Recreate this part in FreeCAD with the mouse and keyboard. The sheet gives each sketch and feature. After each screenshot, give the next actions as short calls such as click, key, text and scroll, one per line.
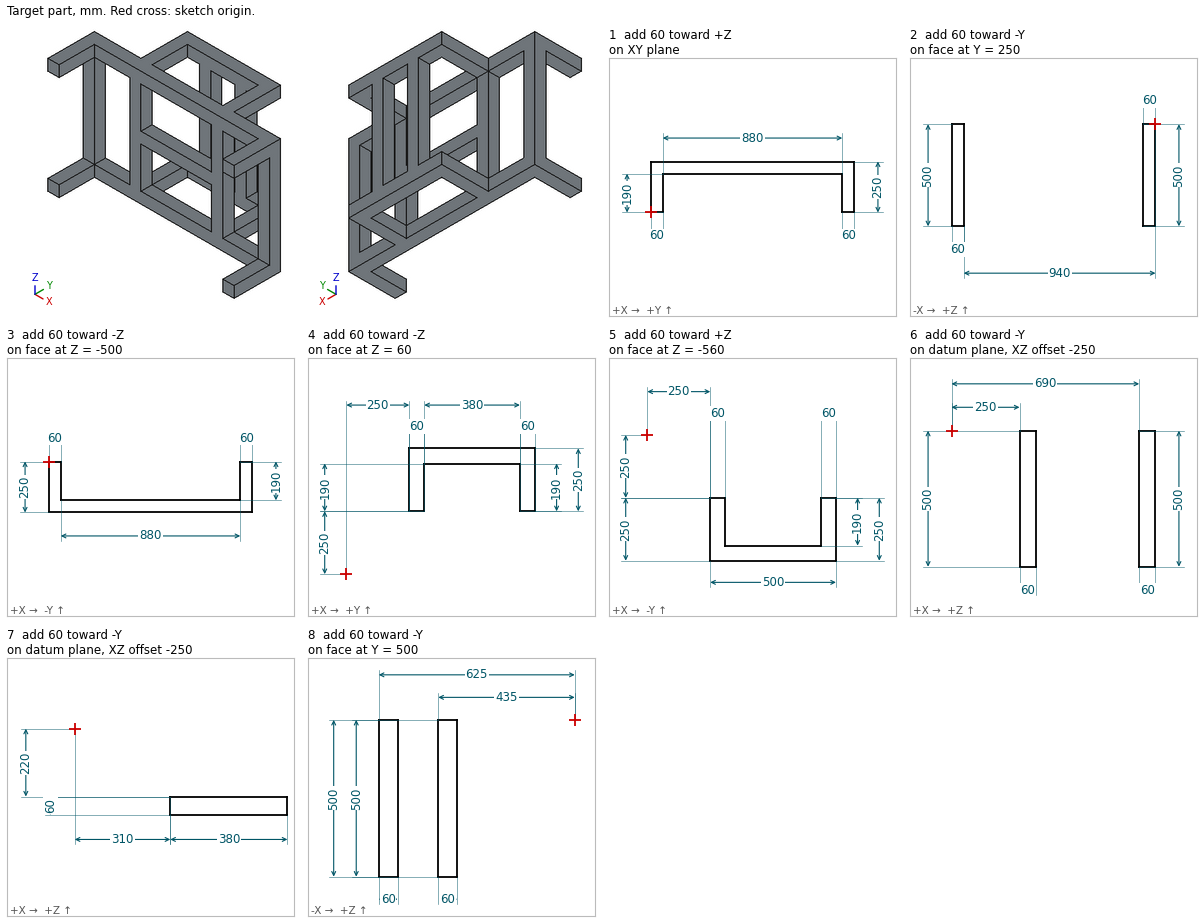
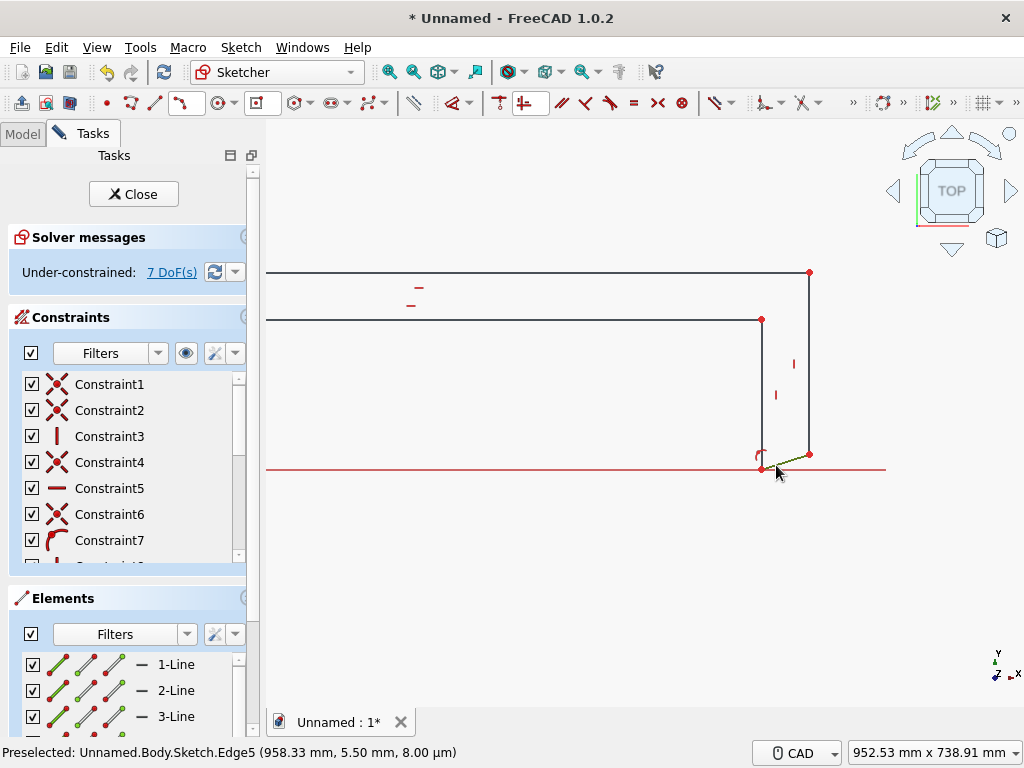
click(544, 104)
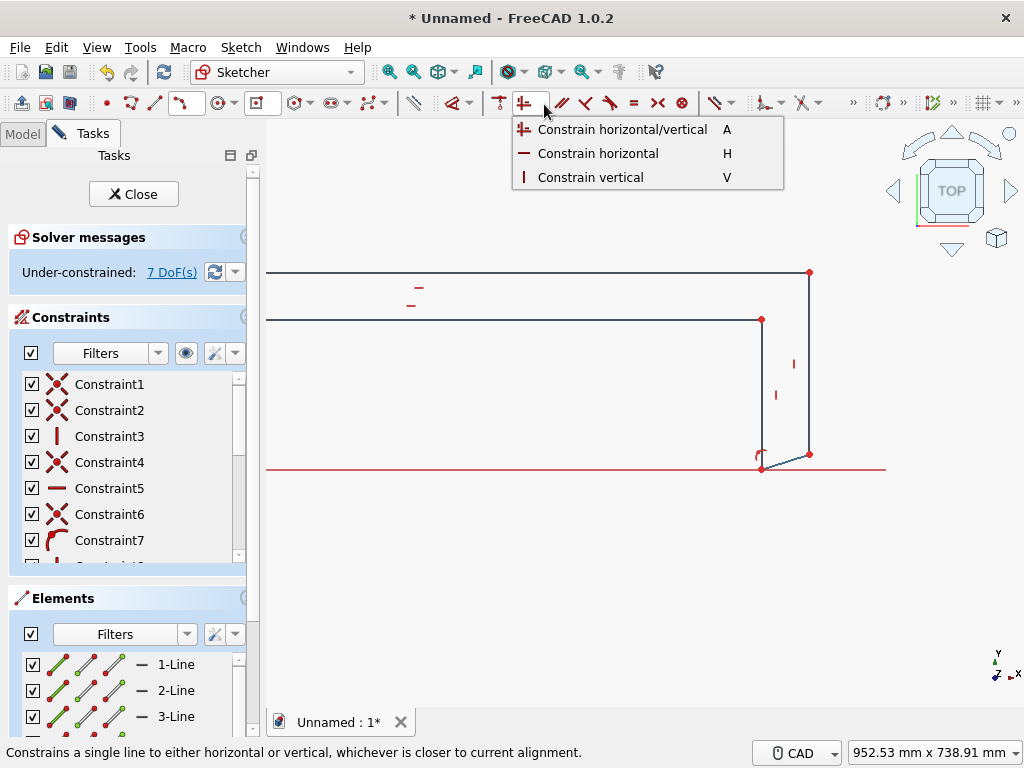
click(648, 153)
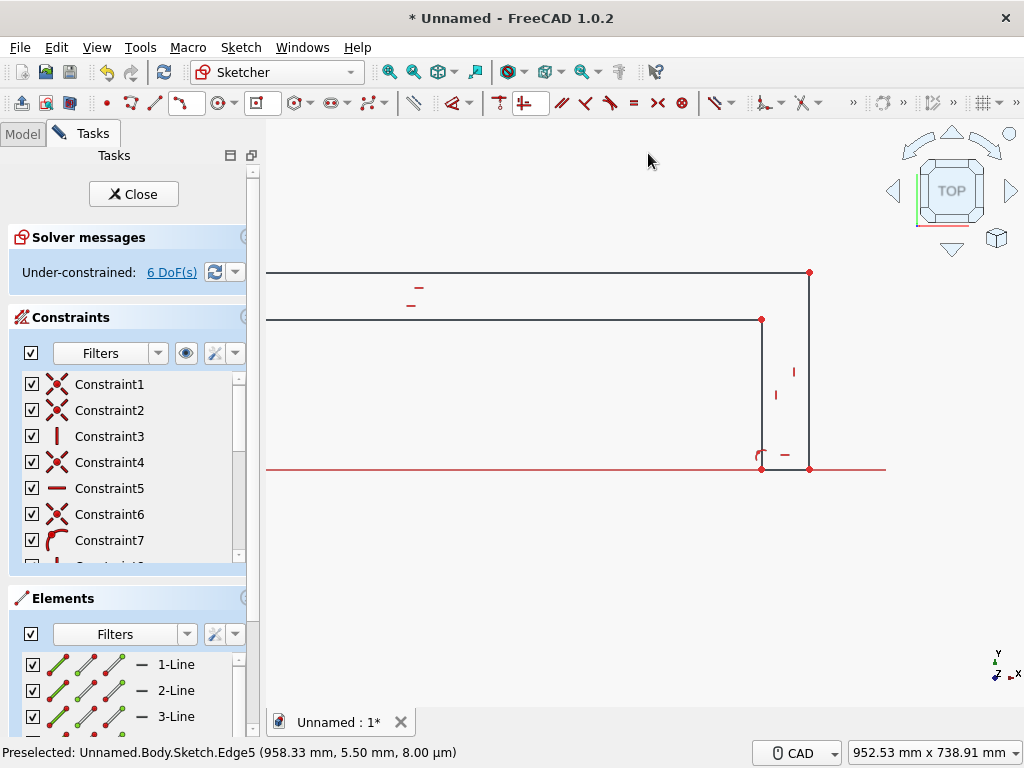
scroll(778, 465, down, 3)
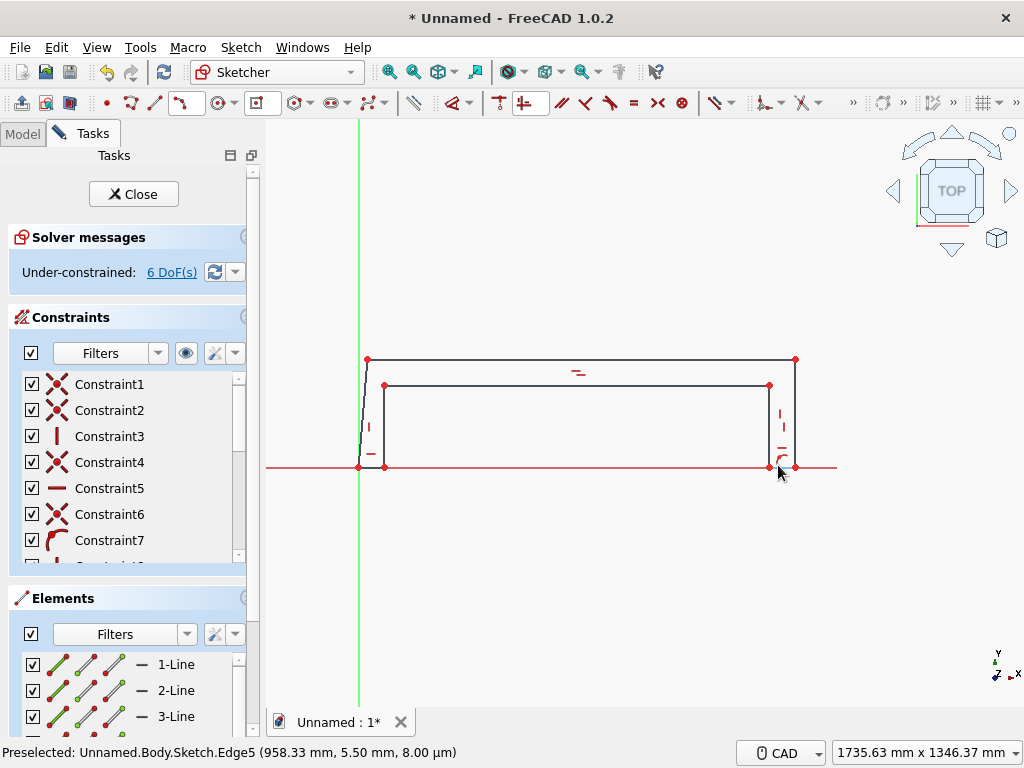
scroll(365, 392, up, 4)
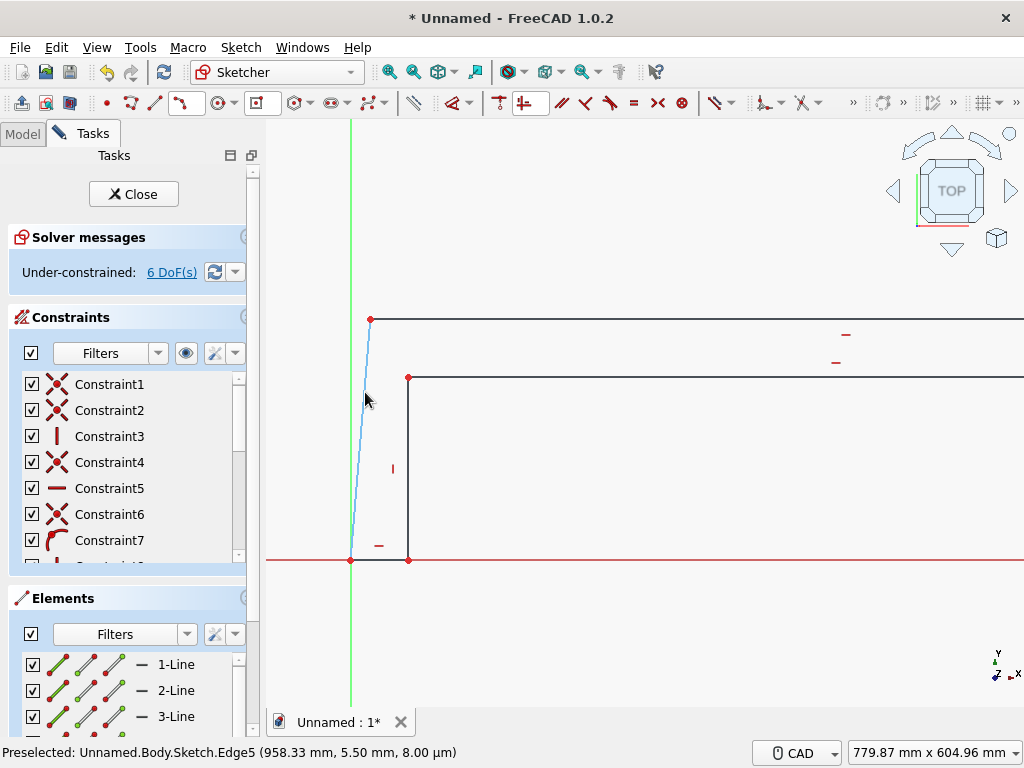
click(364, 392)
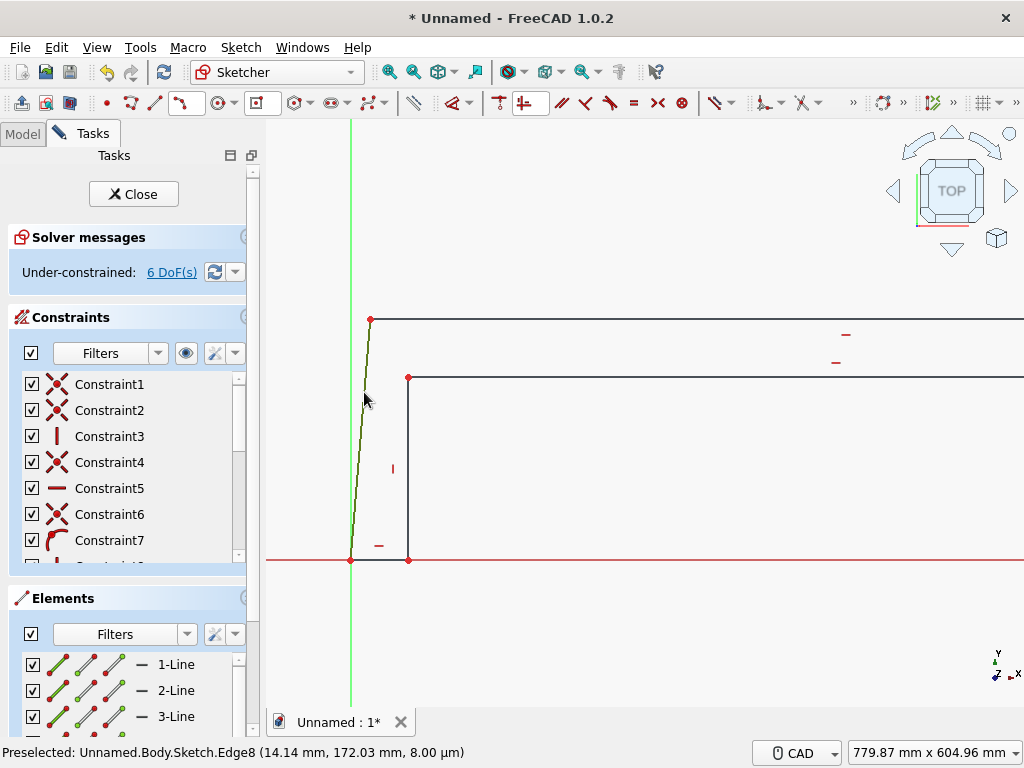
key(v)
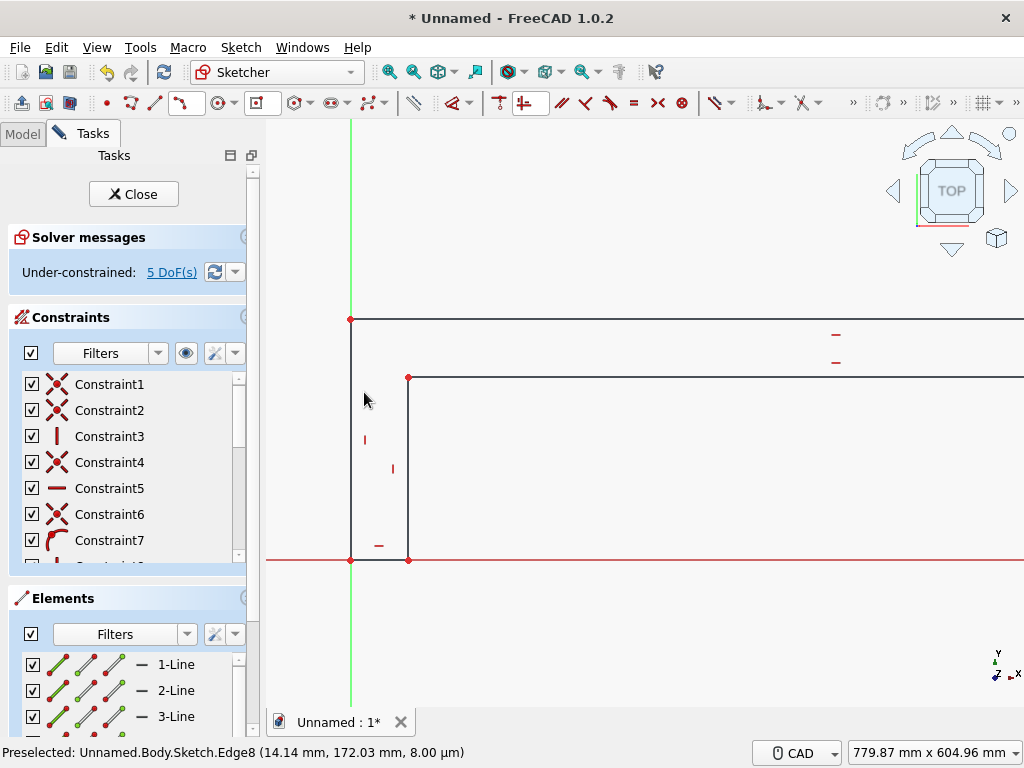
click(452, 104)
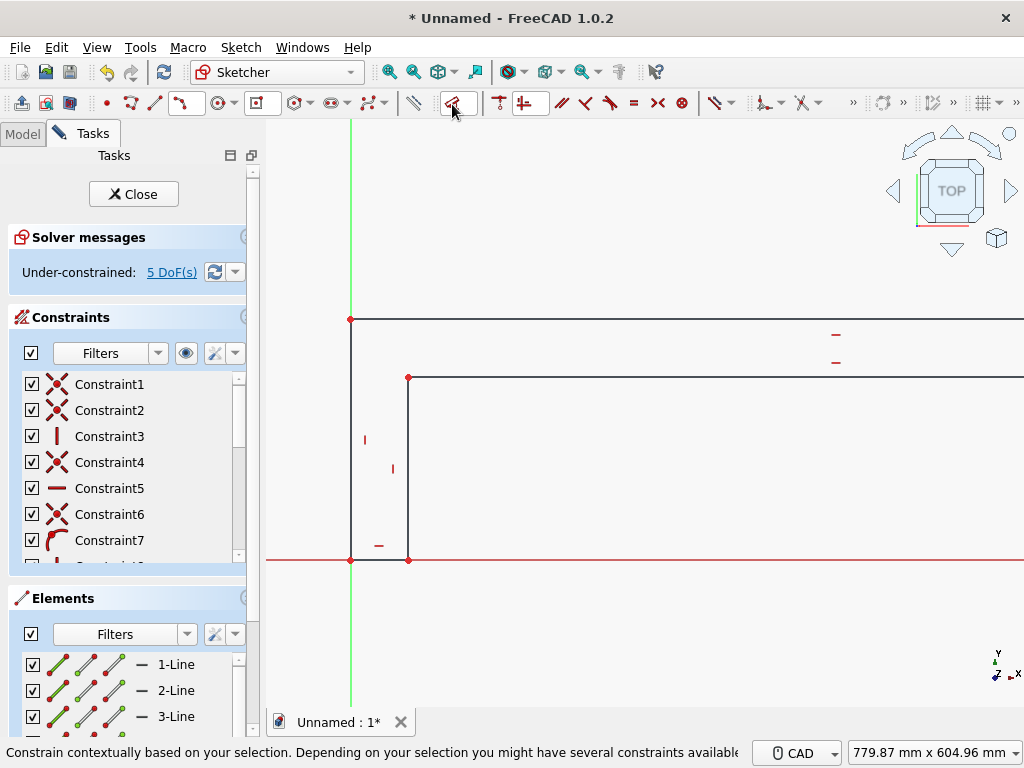
click(368, 560)
click(379, 594)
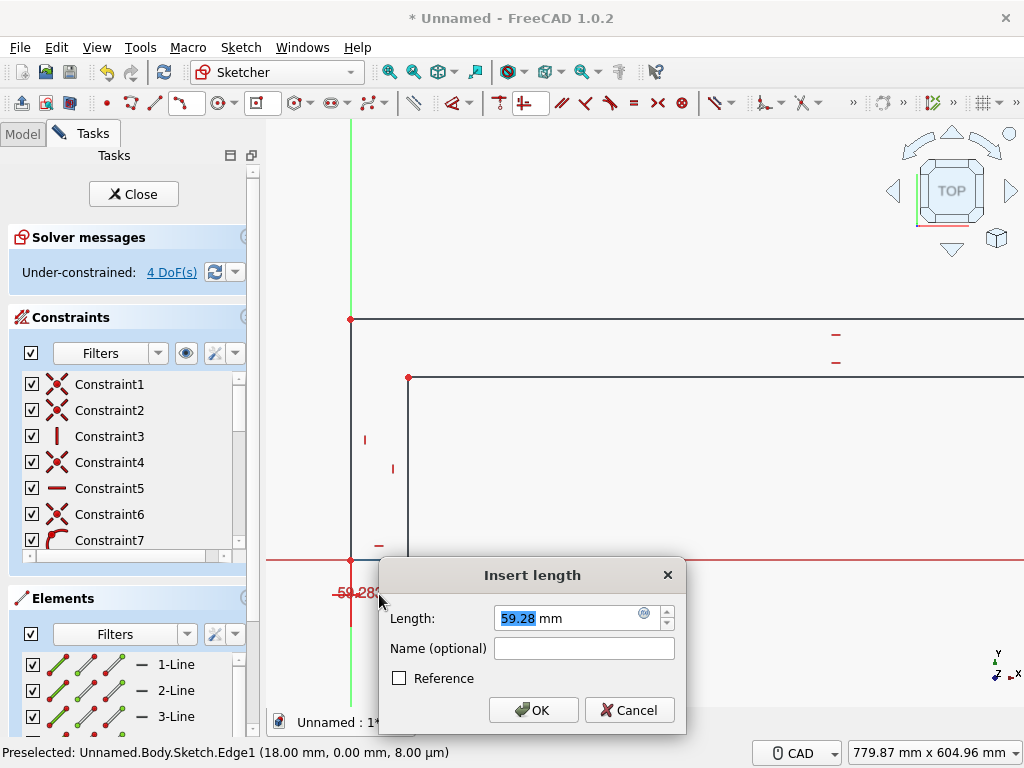
text(60)
key(Return)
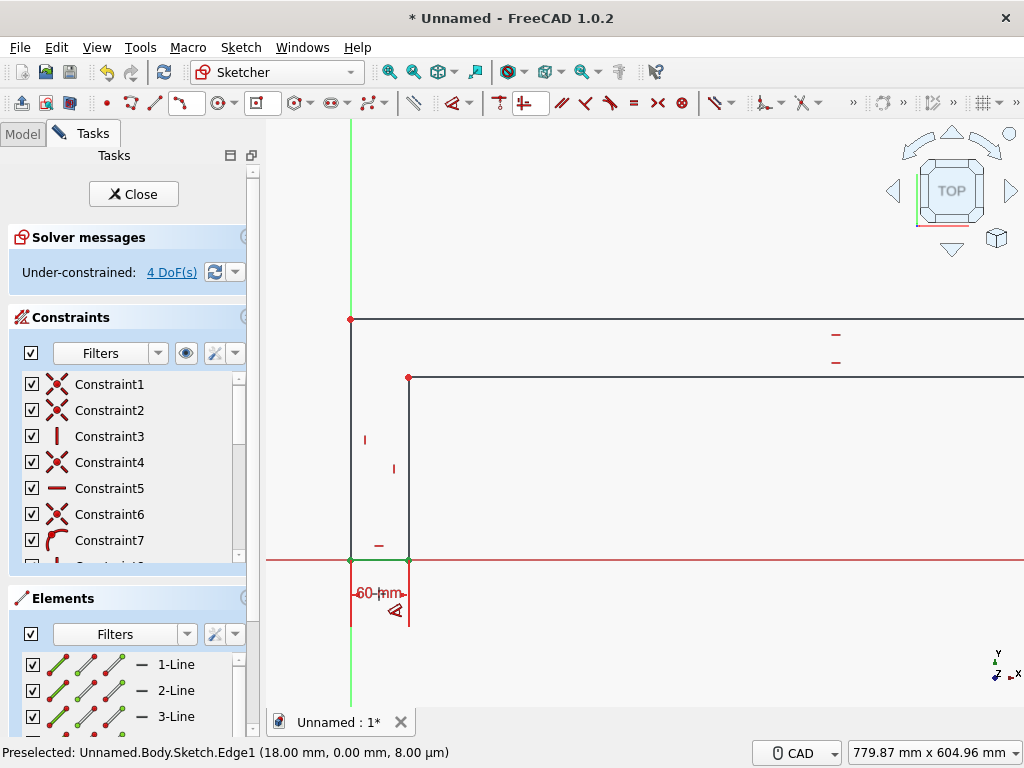
scroll(364, 392, down, 4)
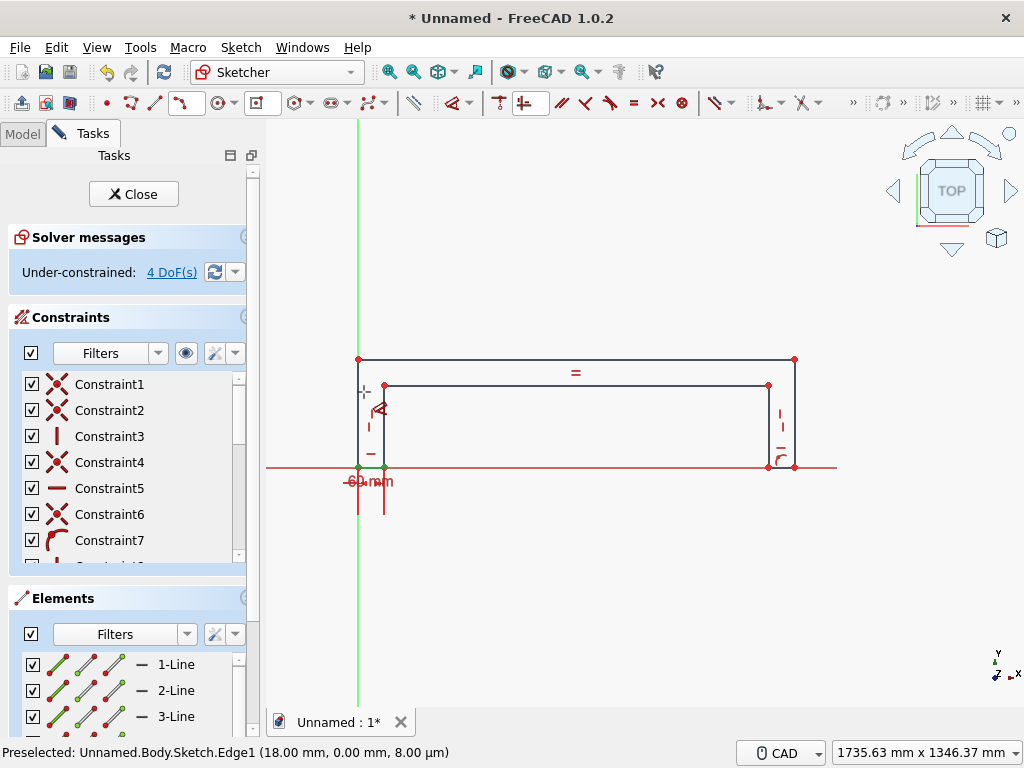
scroll(777, 468, up, 3)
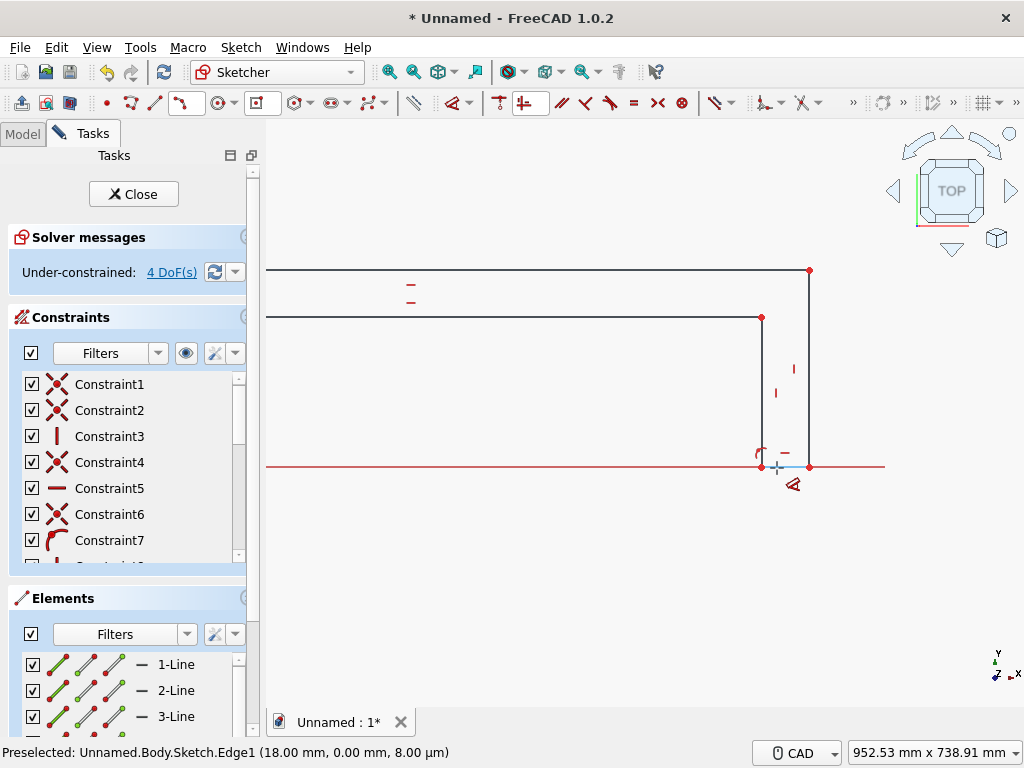
click(776, 467)
click(785, 501)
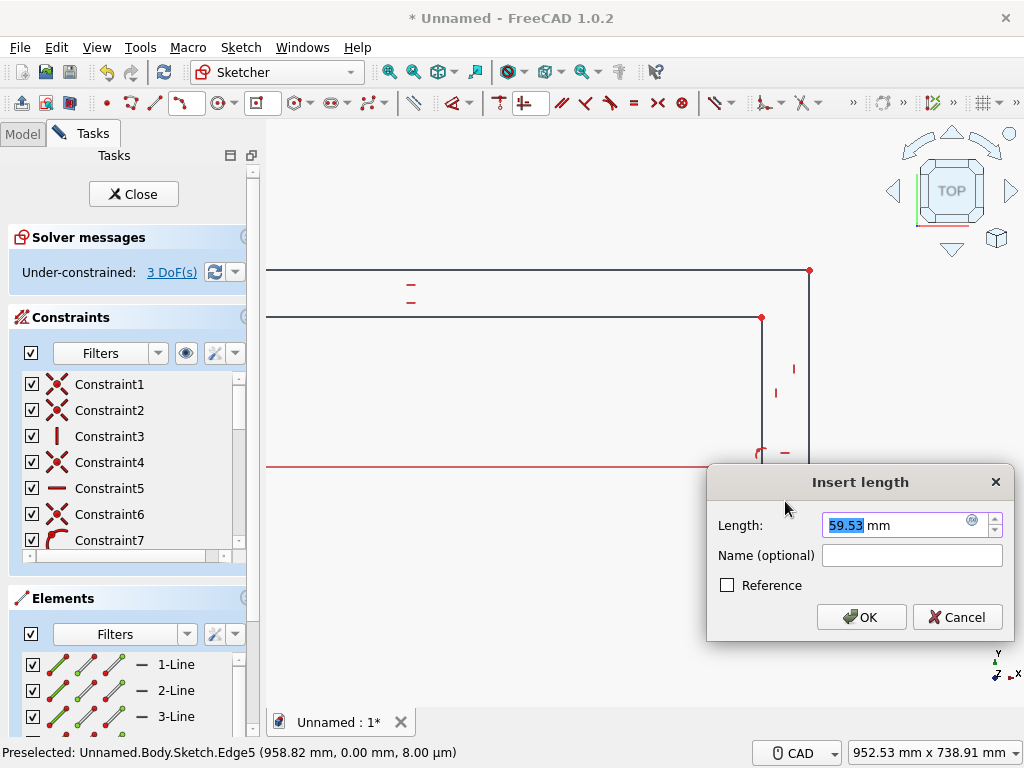
text(60)
key(Return)